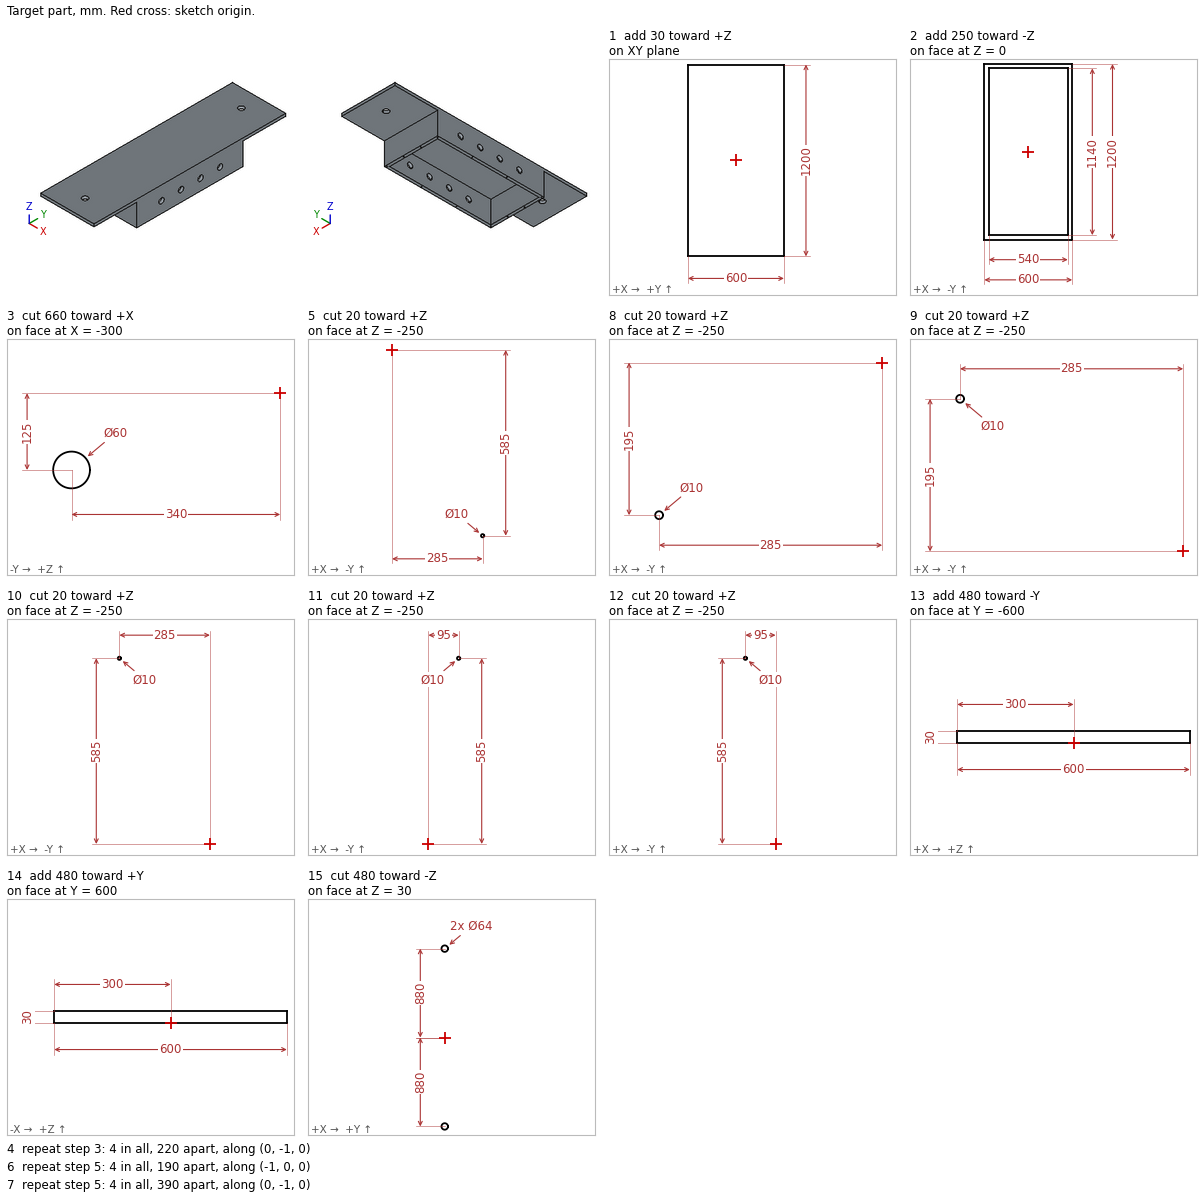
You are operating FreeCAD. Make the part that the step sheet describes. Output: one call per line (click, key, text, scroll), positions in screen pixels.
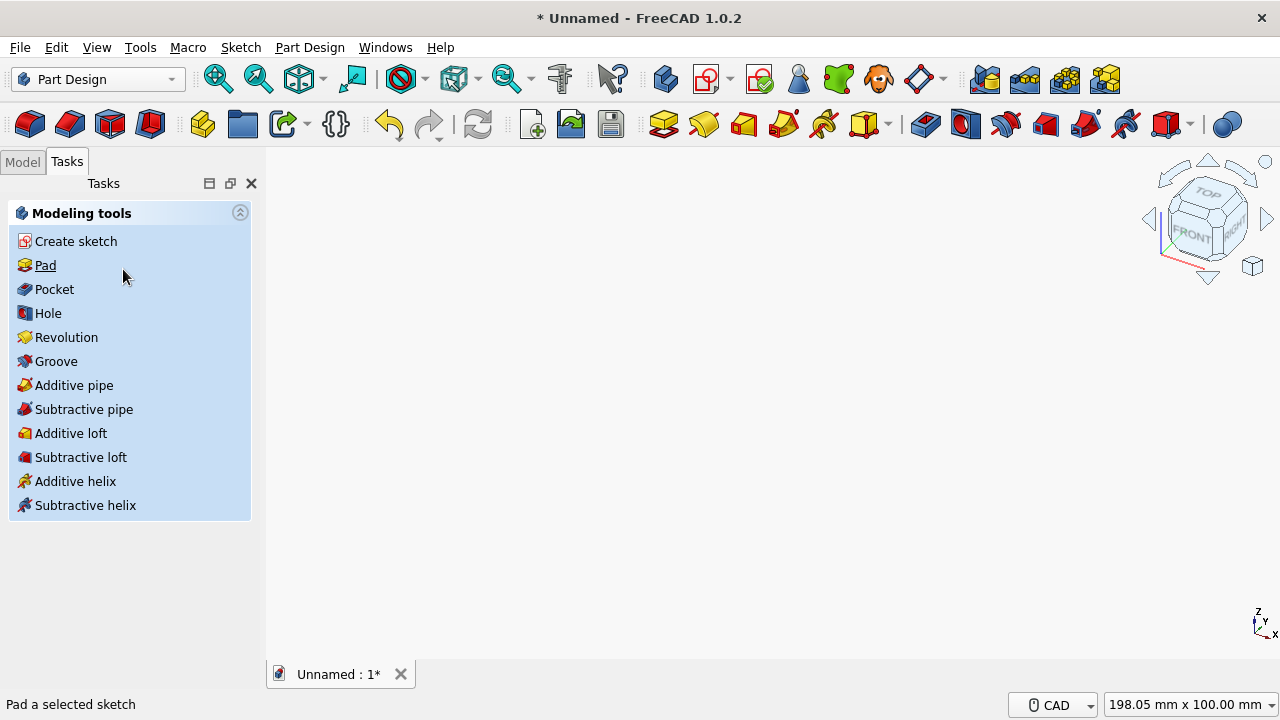
click(664, 124)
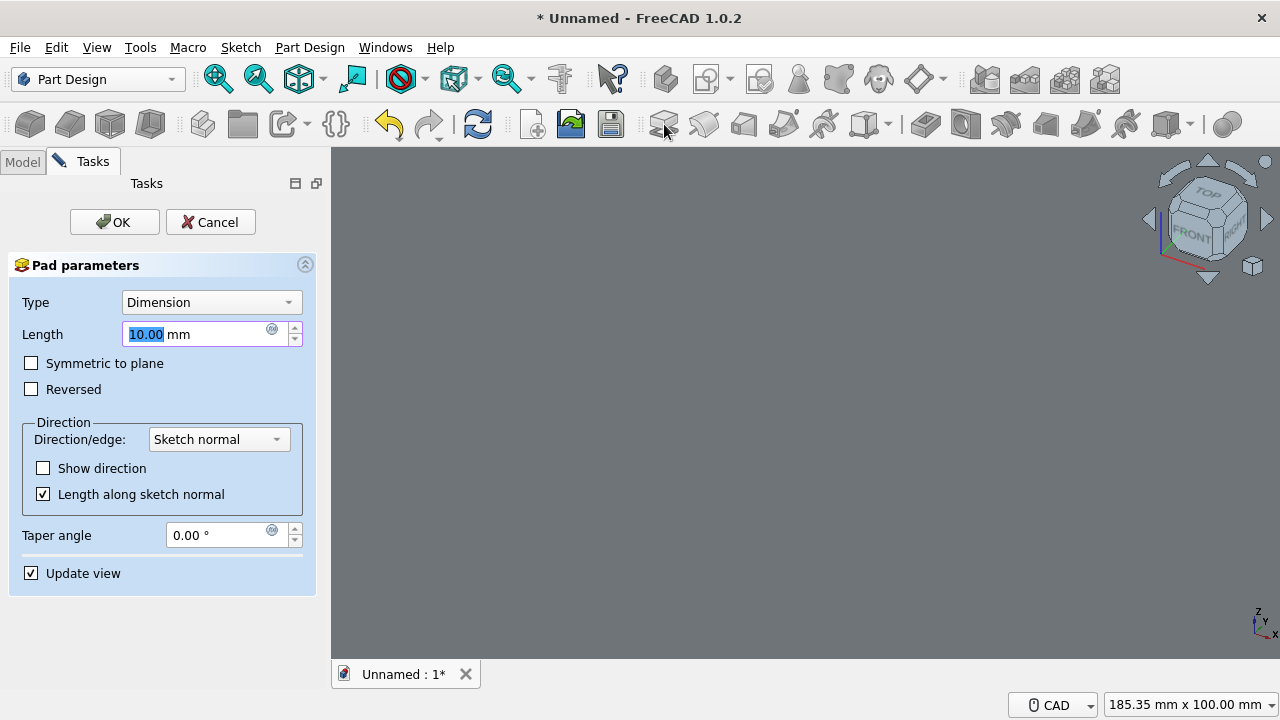
text(30)
key(Tab)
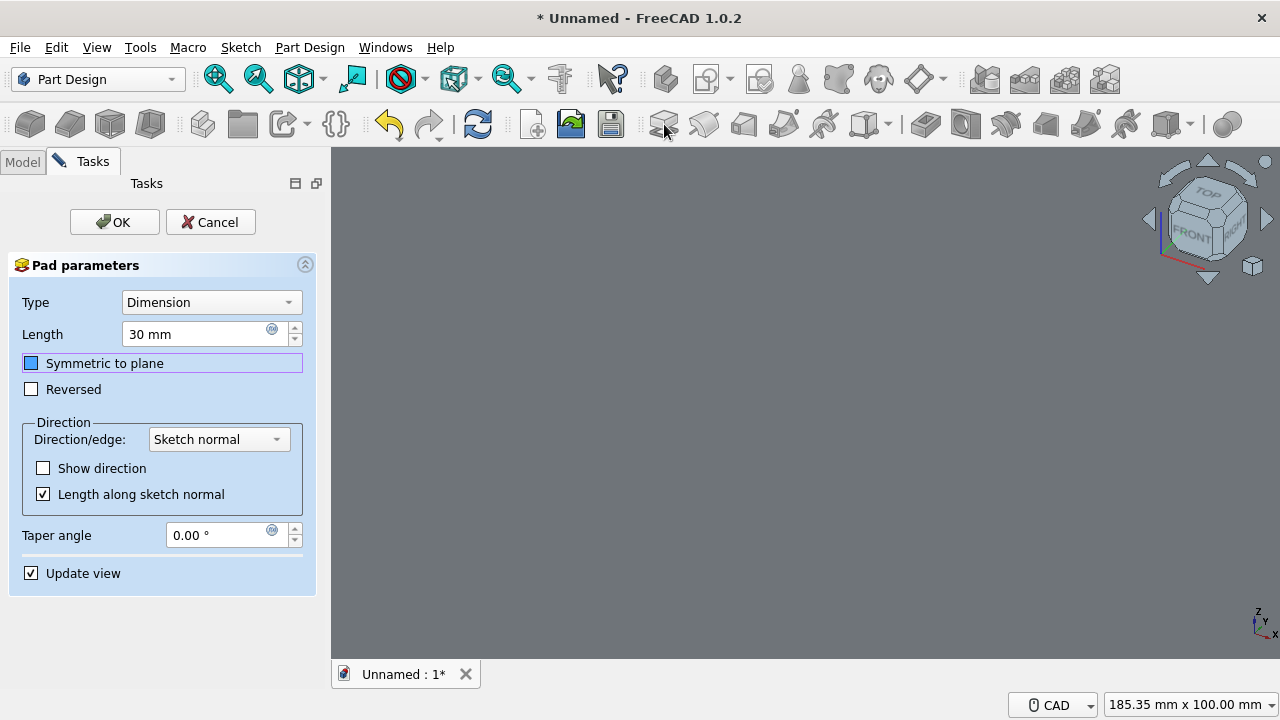
click(115, 222)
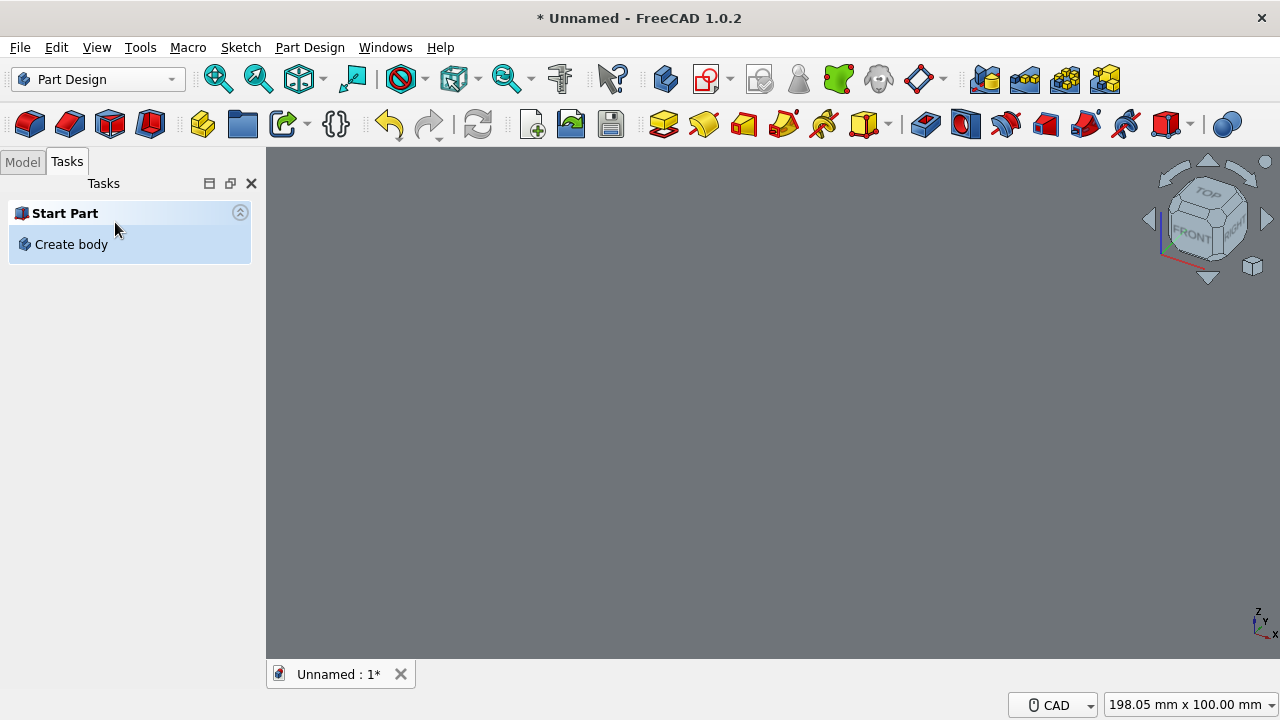
click(220, 80)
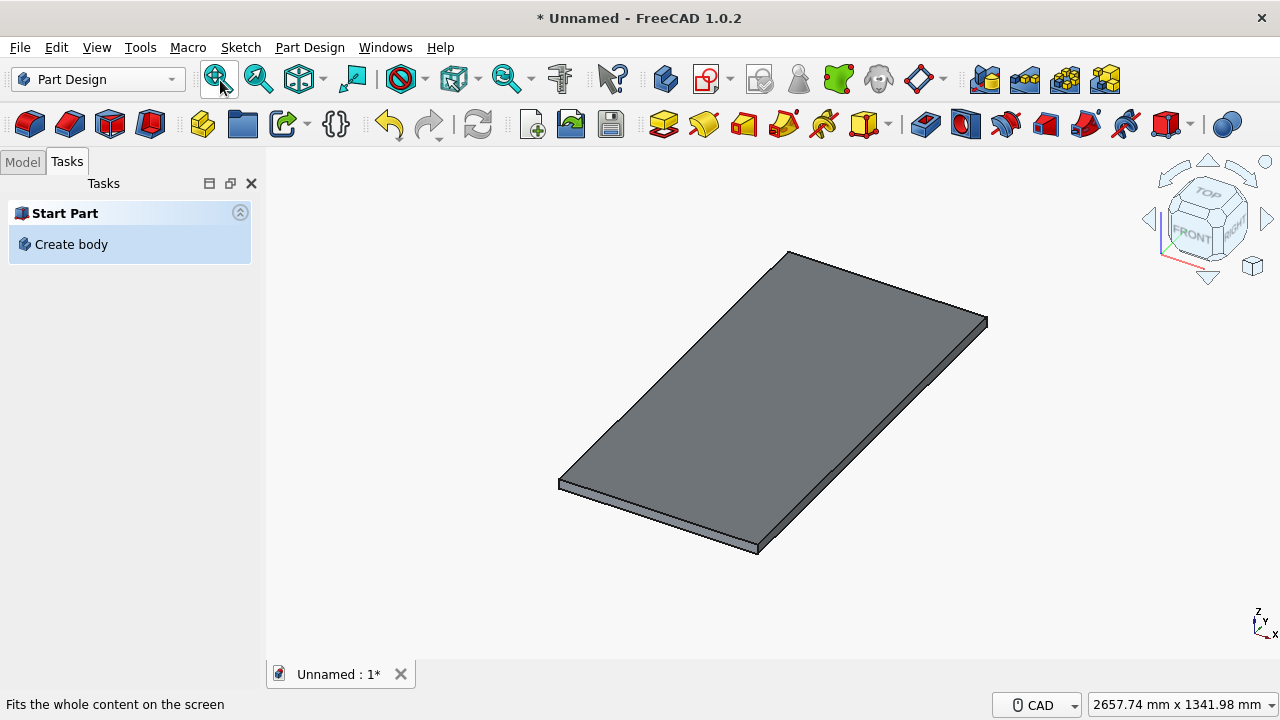
key(5)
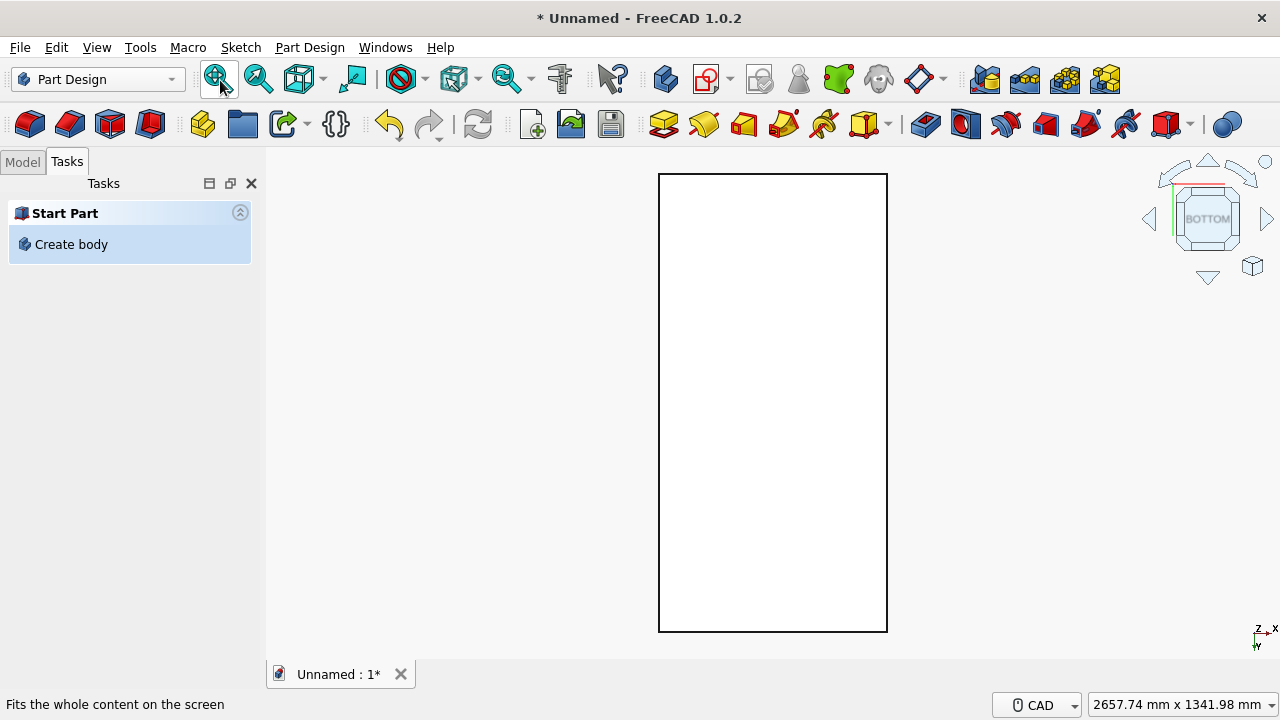
click(773, 467)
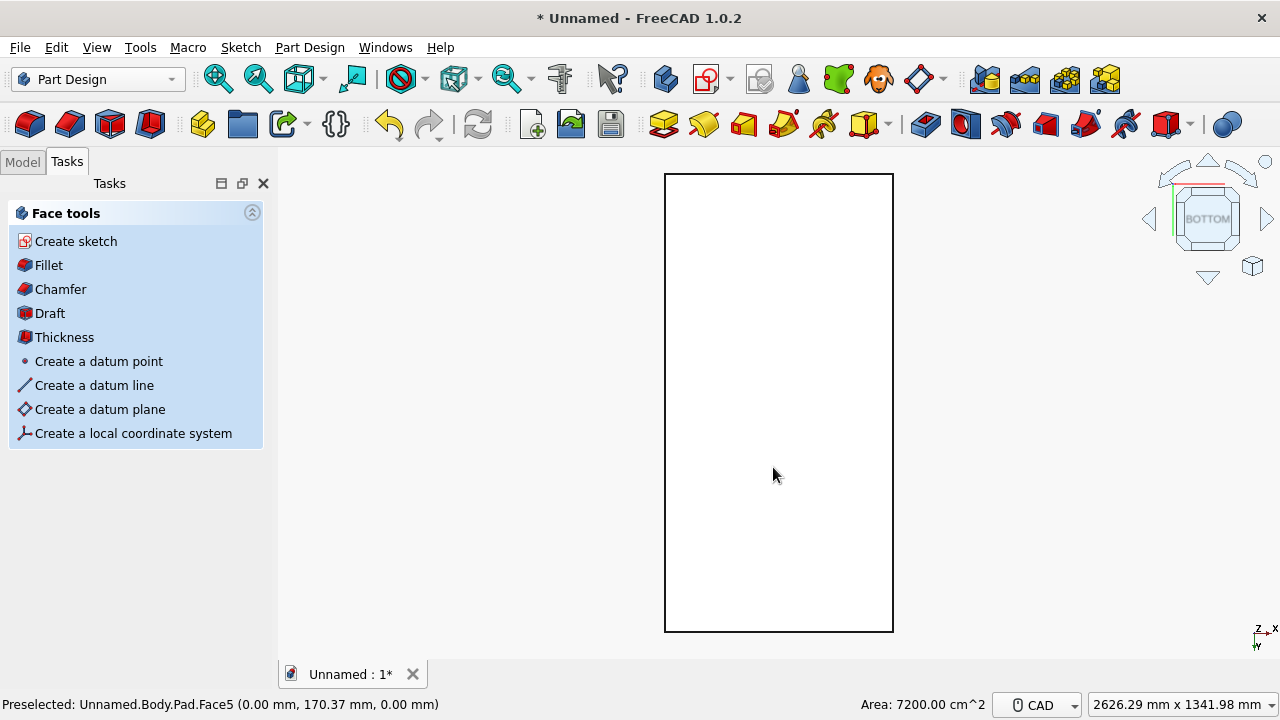
click(706, 80)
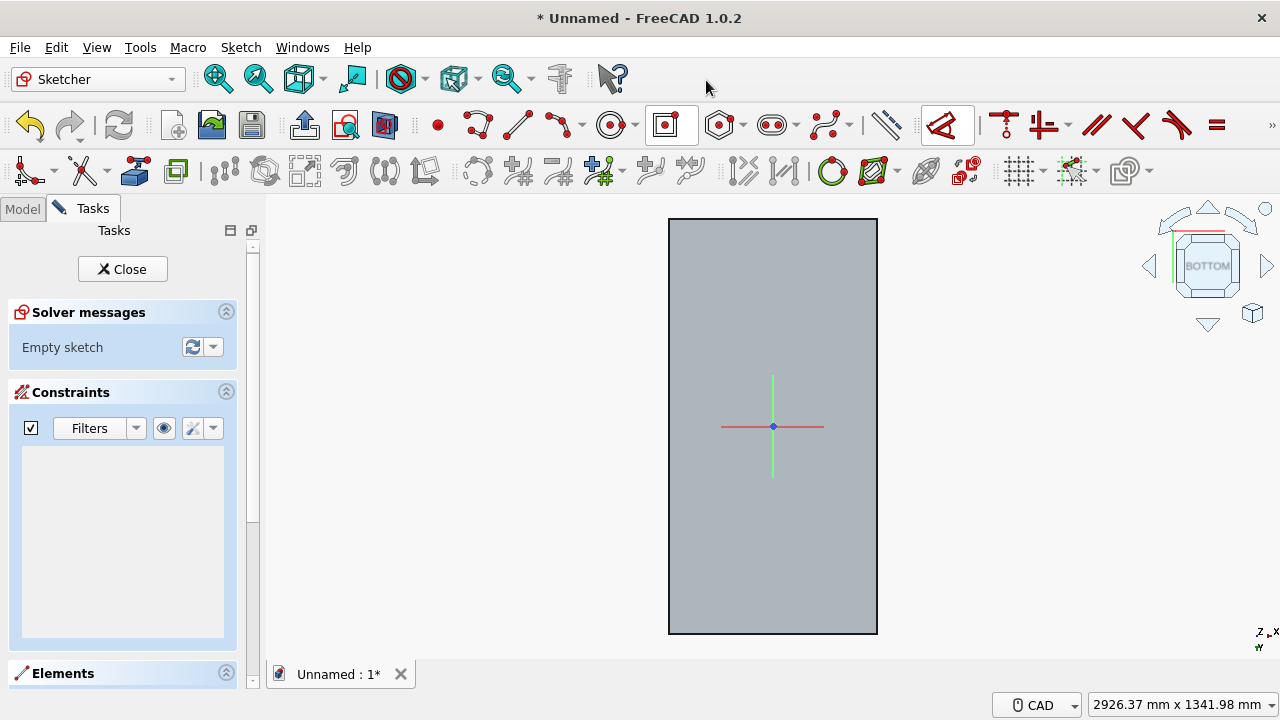
scroll(565, 427, down, 2)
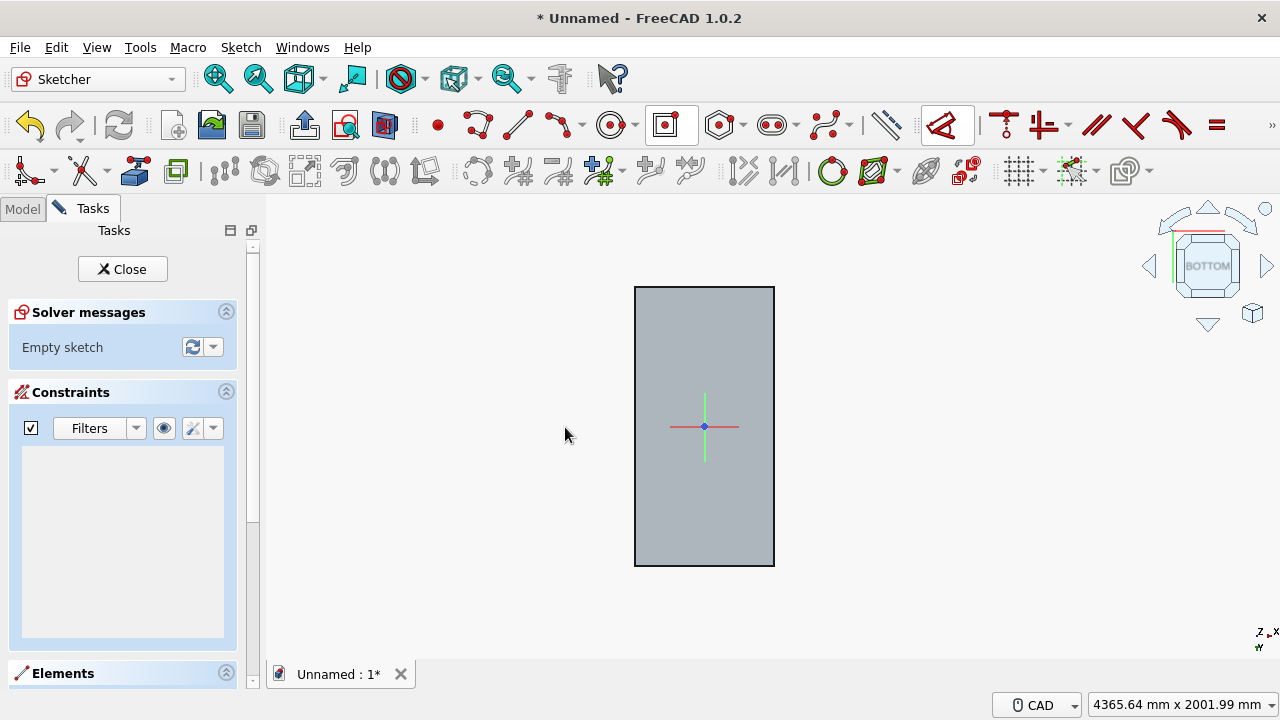
click(666, 126)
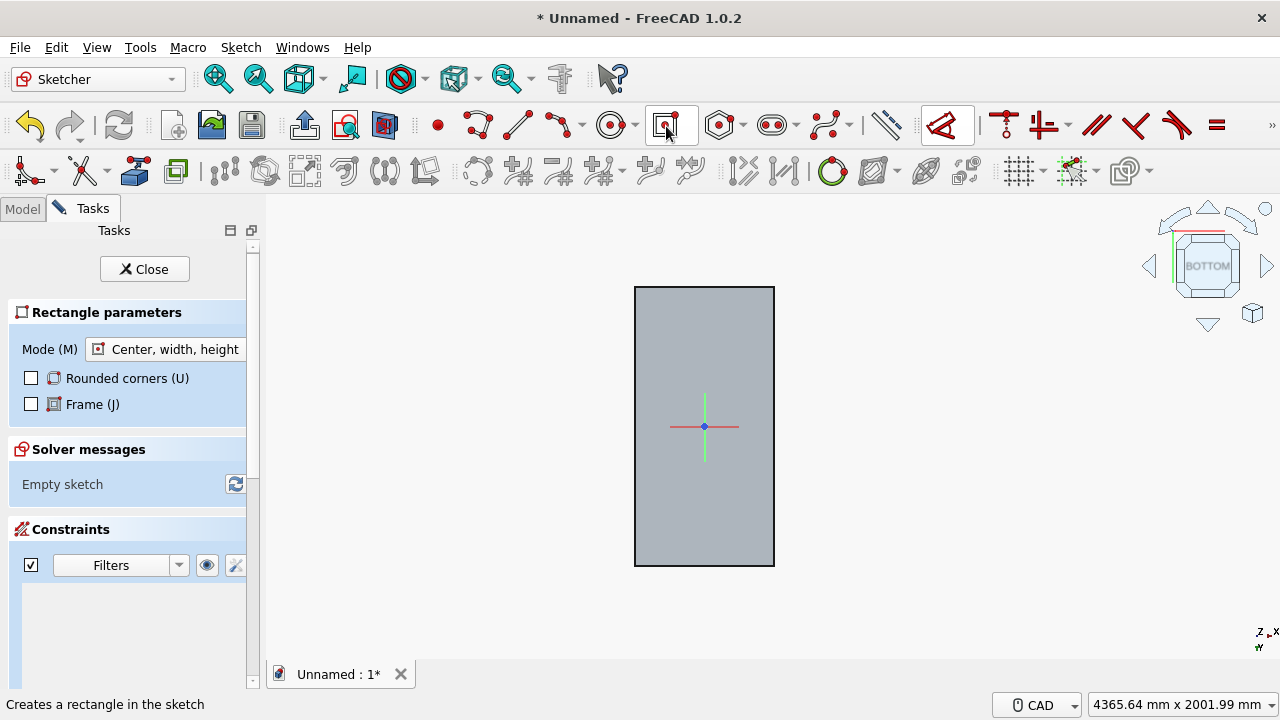
click(705, 427)
move(774, 287)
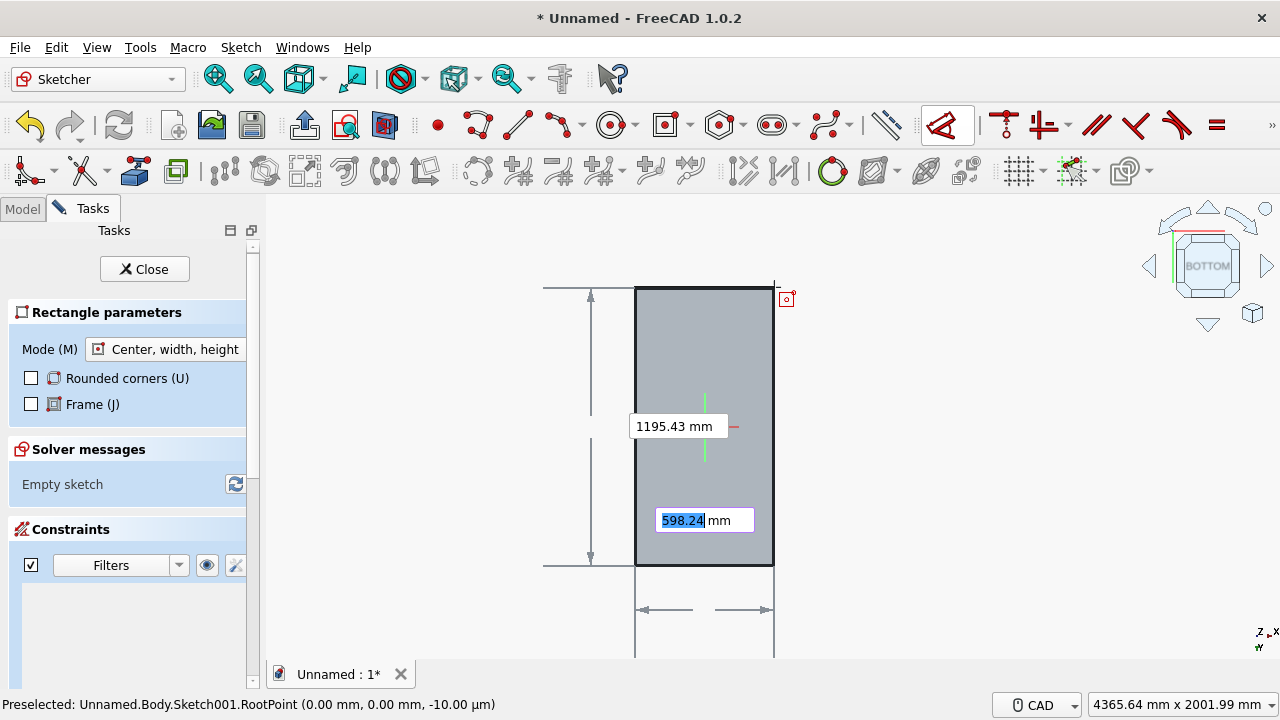
text(600)
key(Tab)
text(1200)
key(Return)